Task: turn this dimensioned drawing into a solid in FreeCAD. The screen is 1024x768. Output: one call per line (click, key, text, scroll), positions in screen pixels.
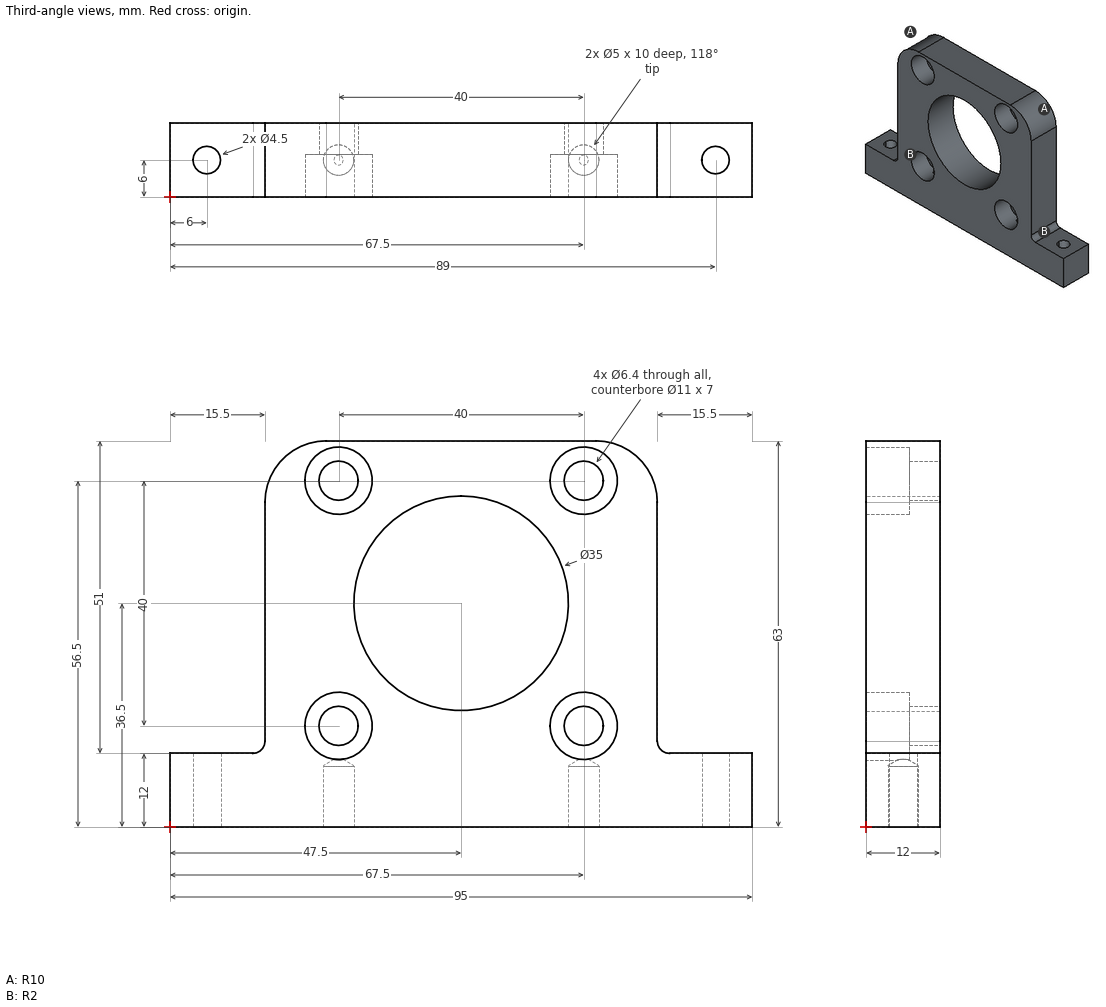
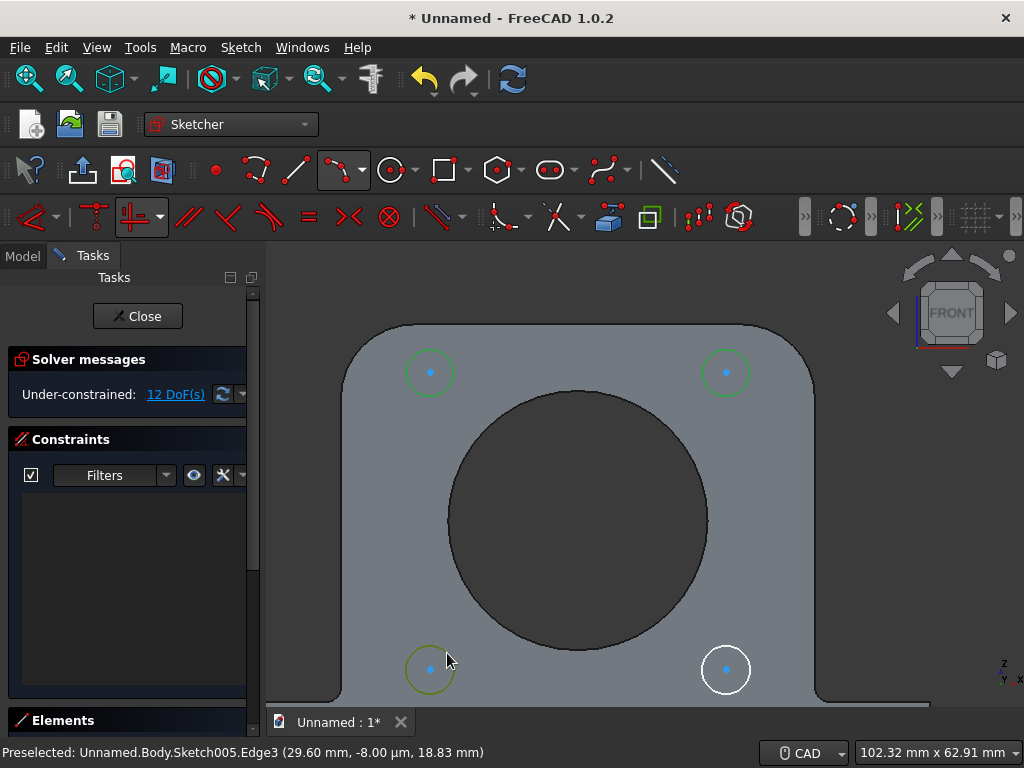
click(743, 653)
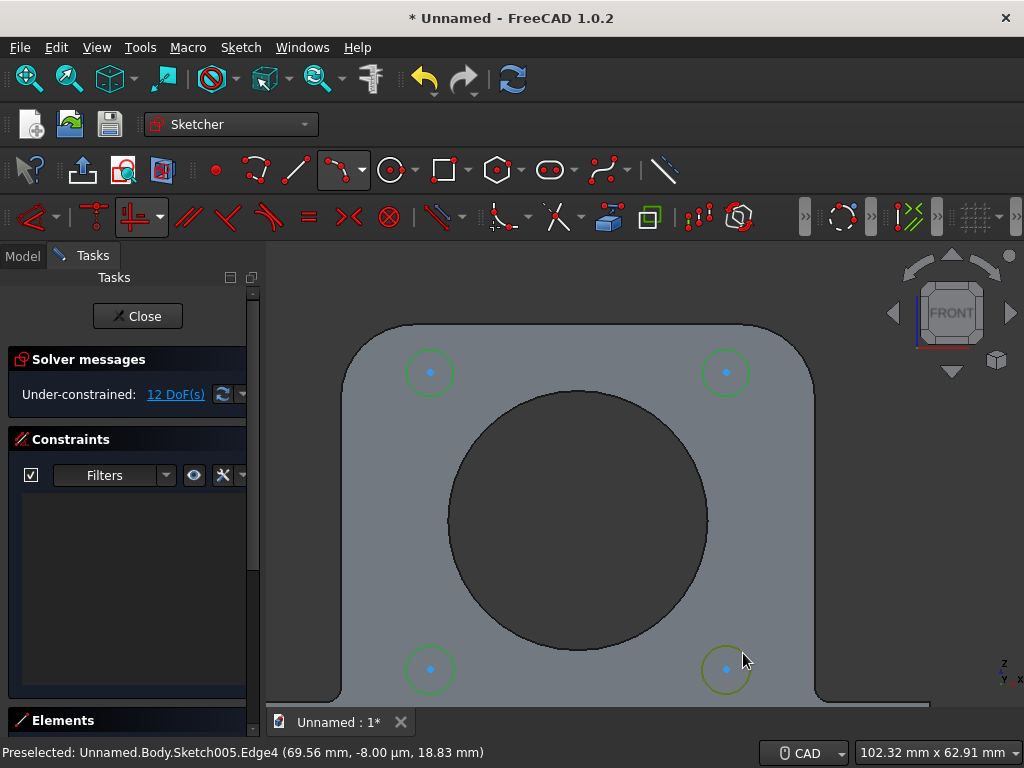
click(310, 218)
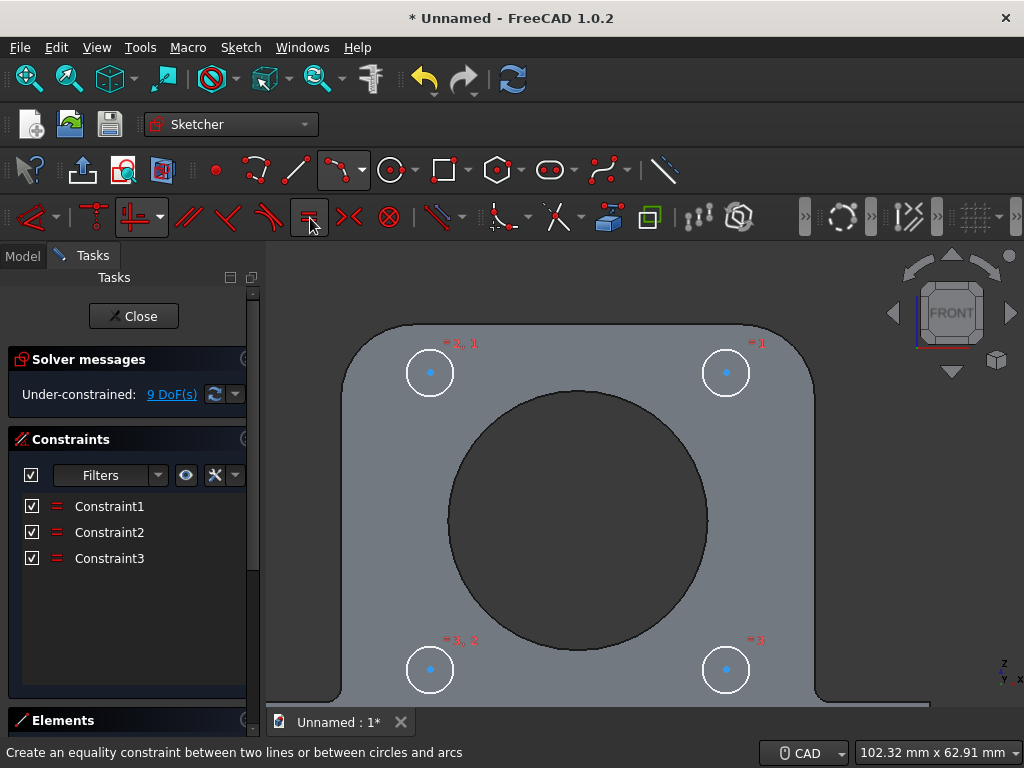
click(726, 373)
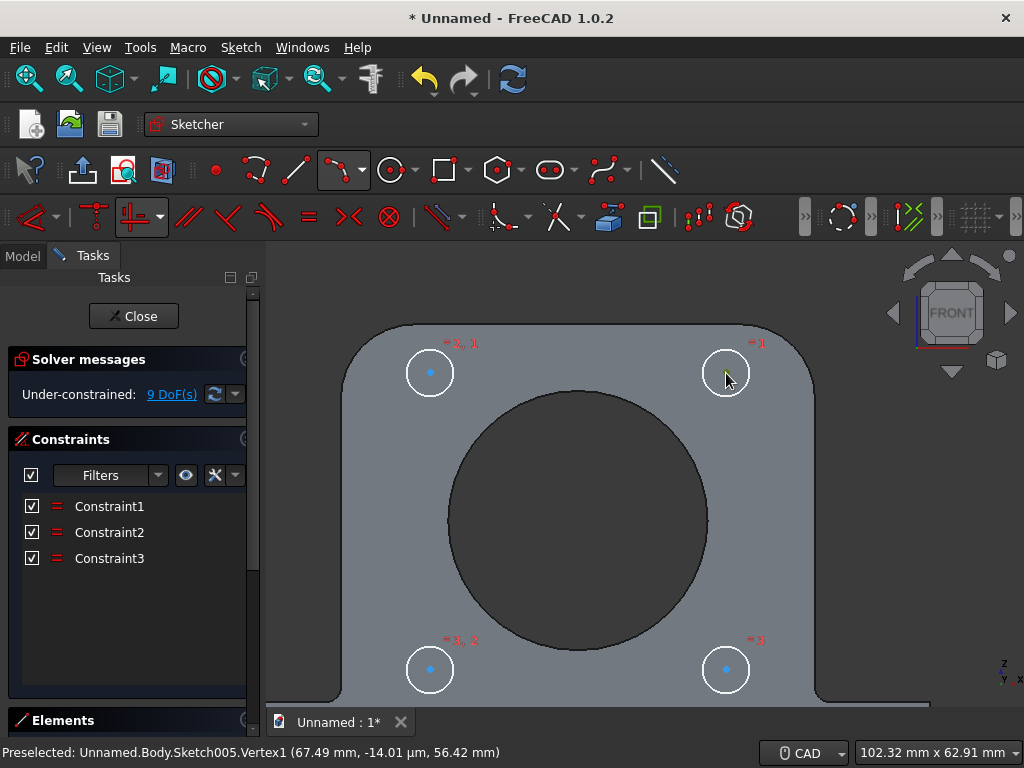
click(430, 373)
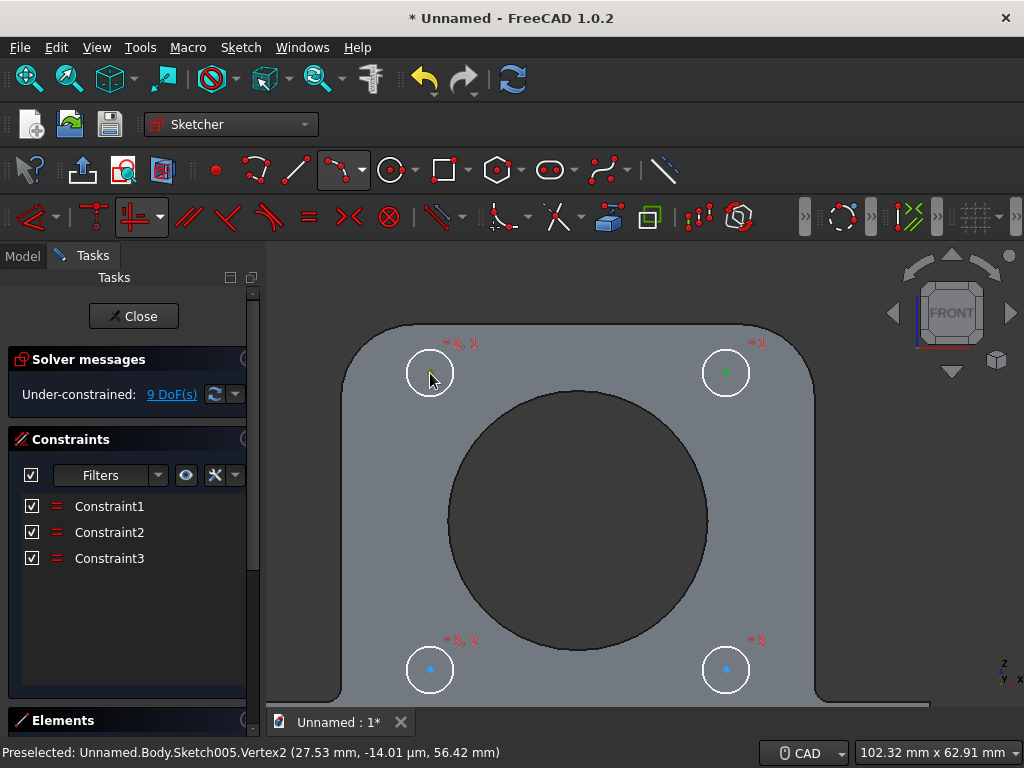
key(h)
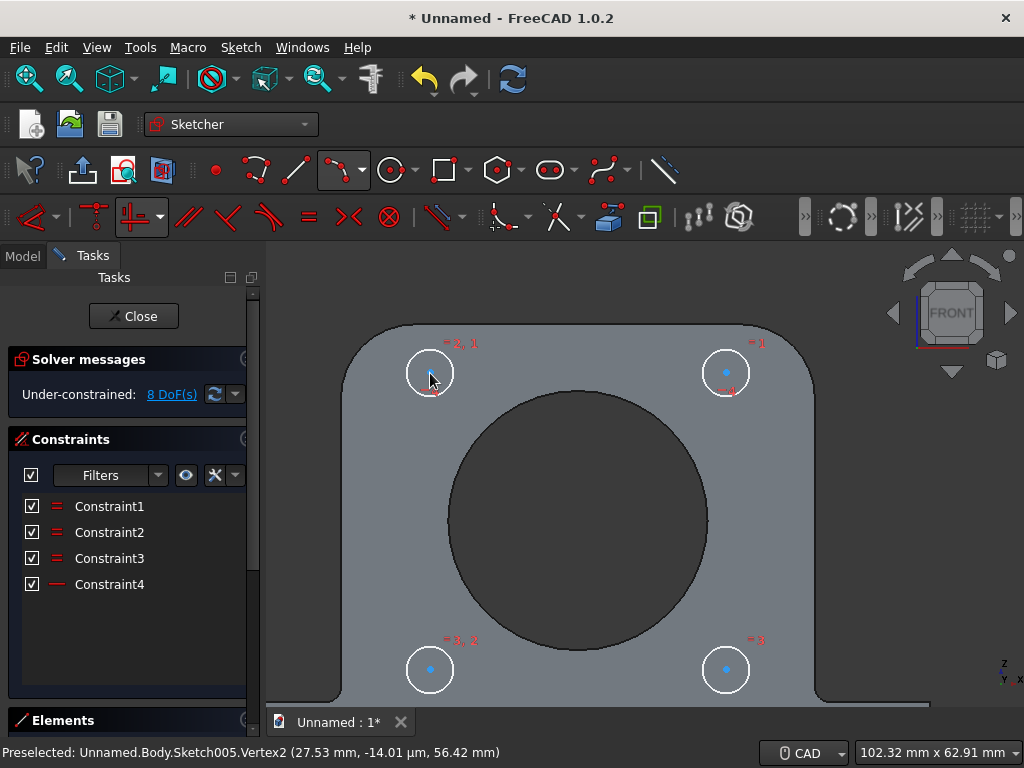
click(430, 373)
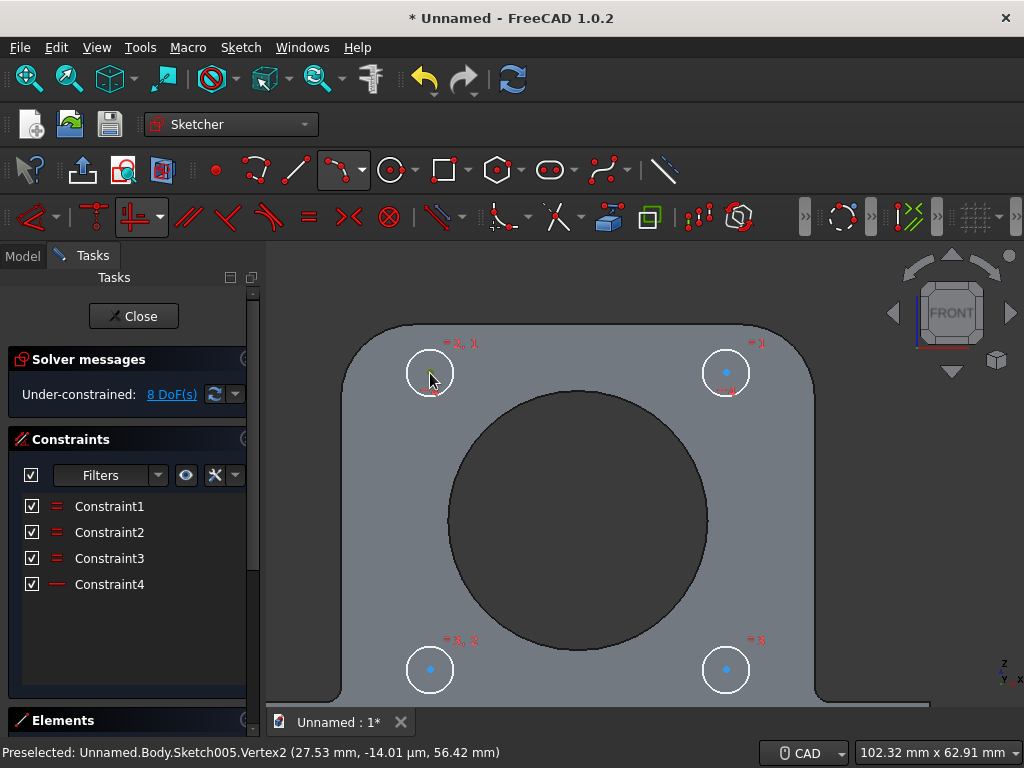
click(430, 670)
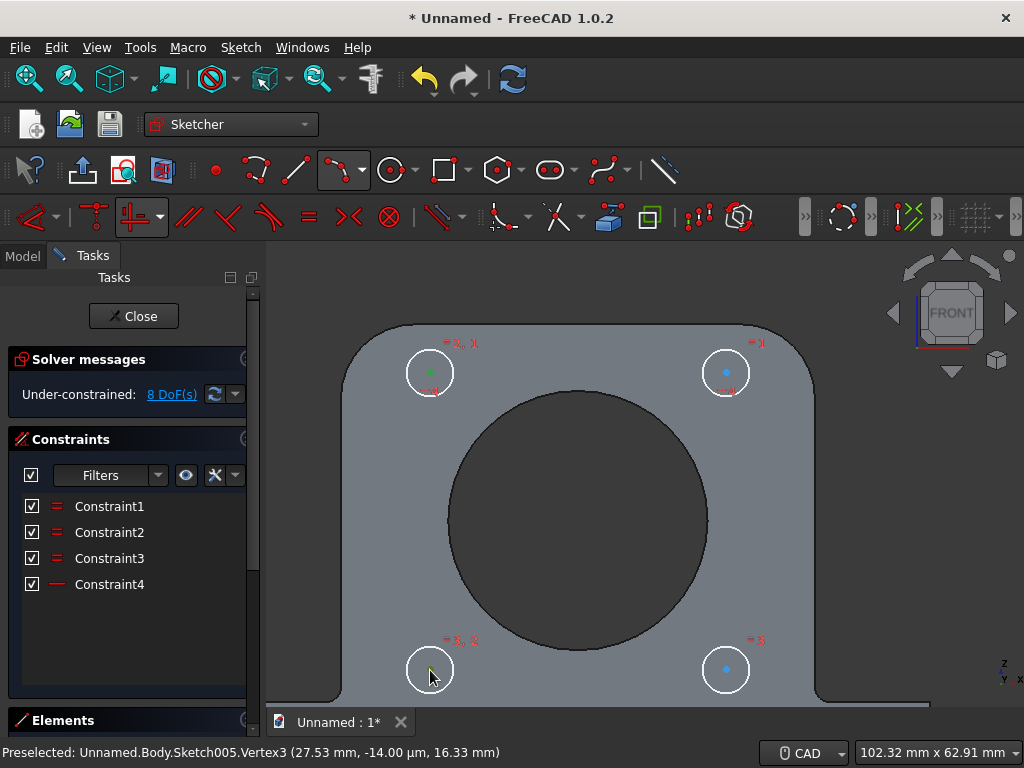
click(162, 218)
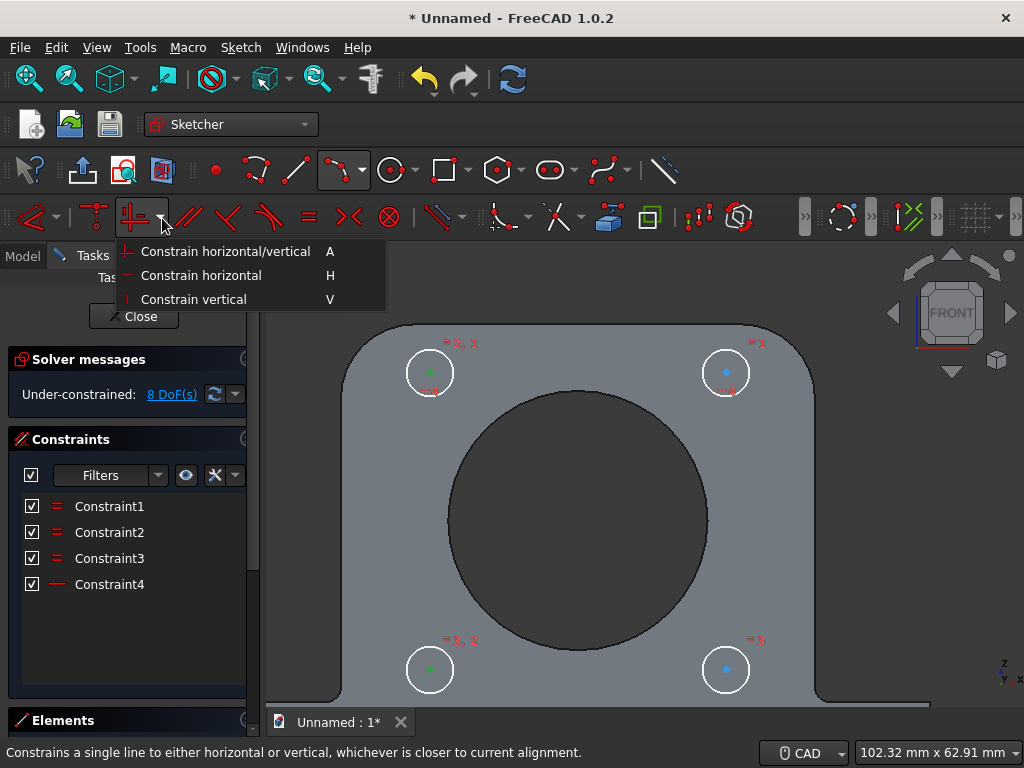
click(251, 299)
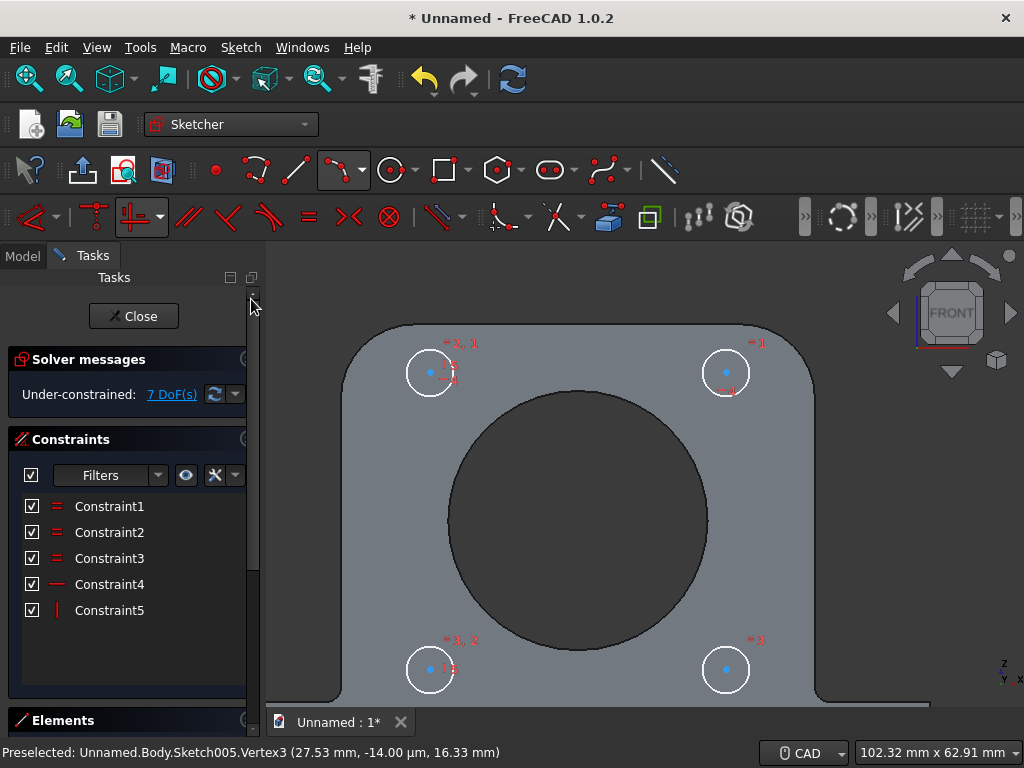
click(726, 373)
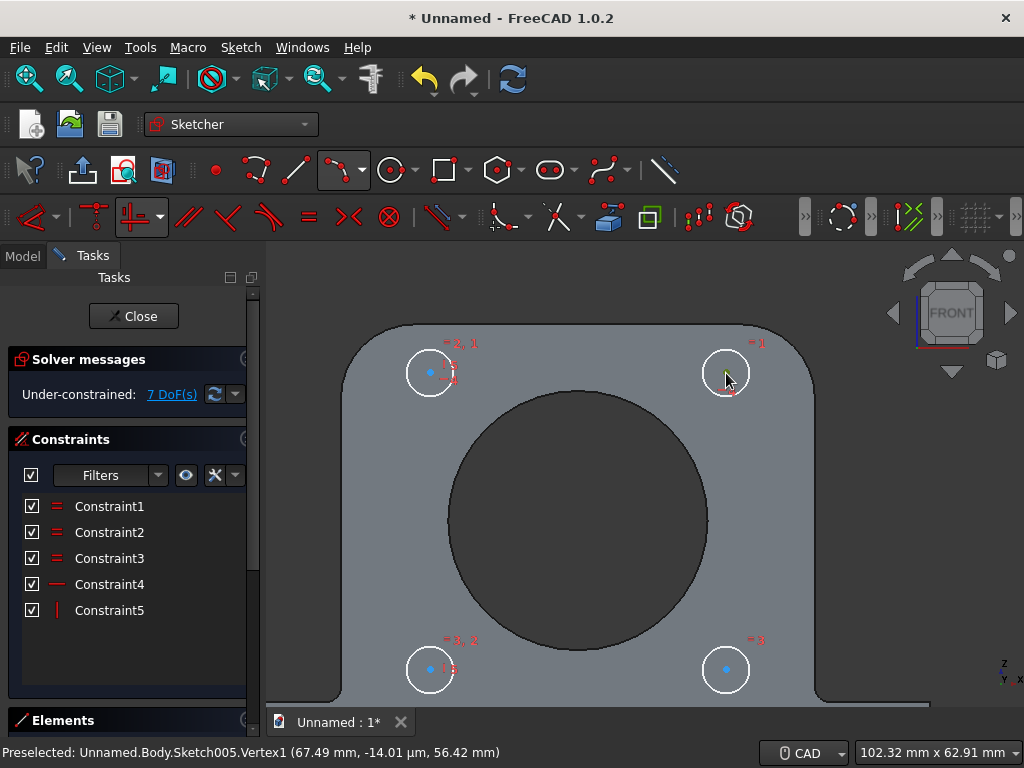
click(726, 670)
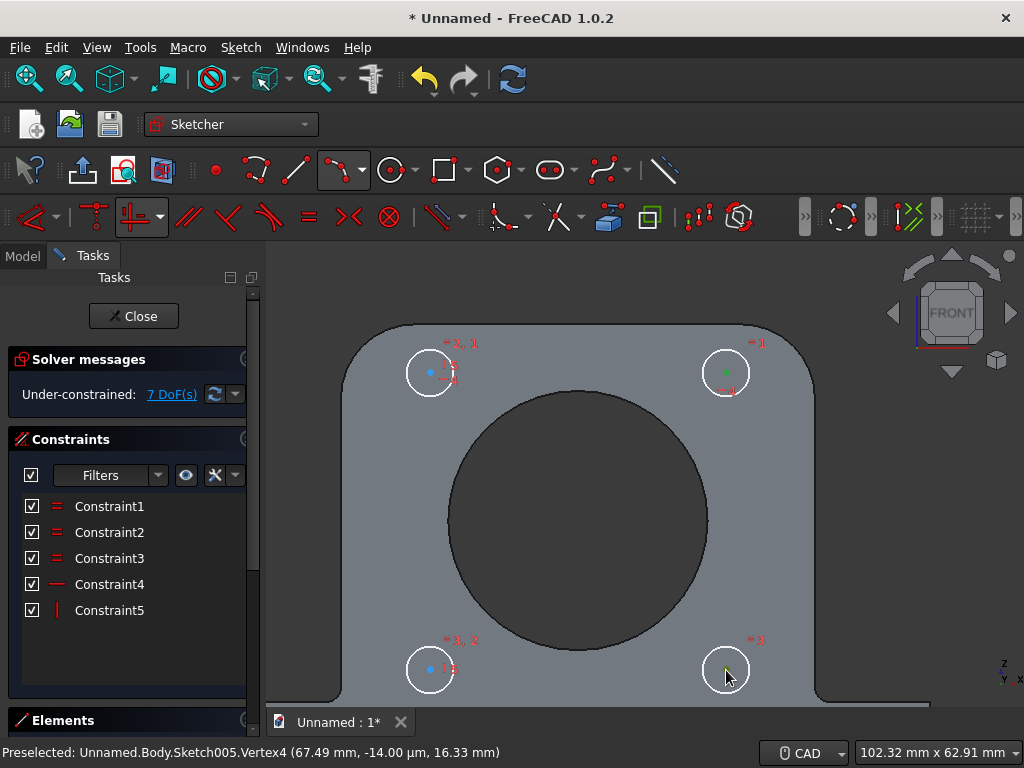
key(v)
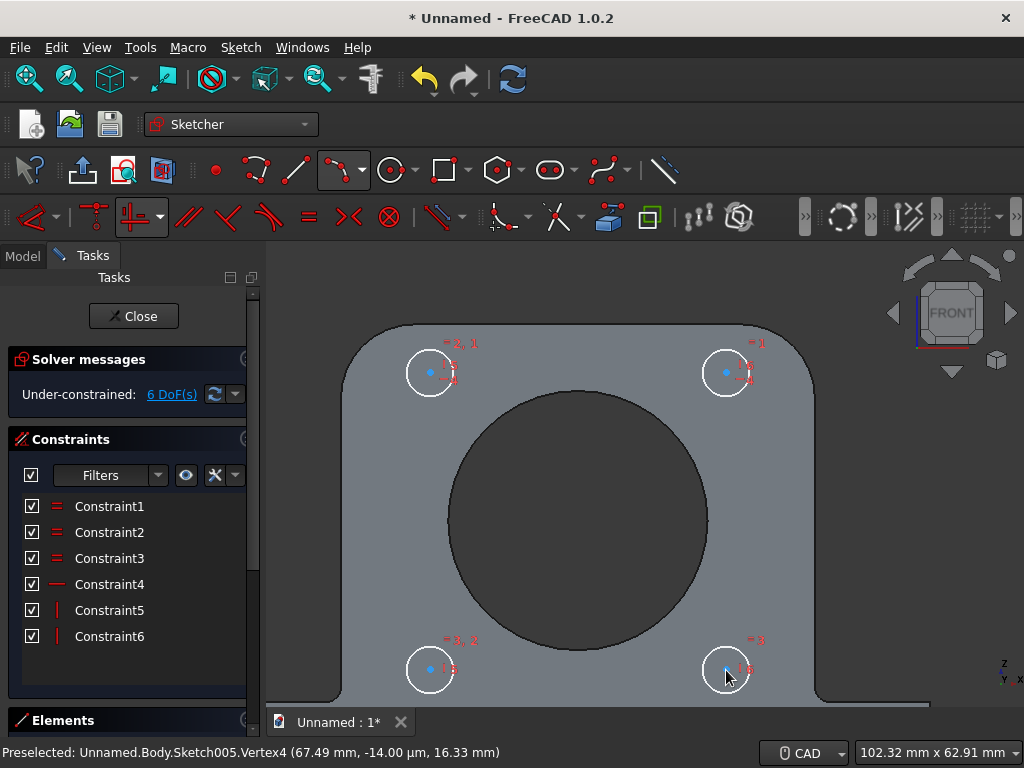
click(430, 670)